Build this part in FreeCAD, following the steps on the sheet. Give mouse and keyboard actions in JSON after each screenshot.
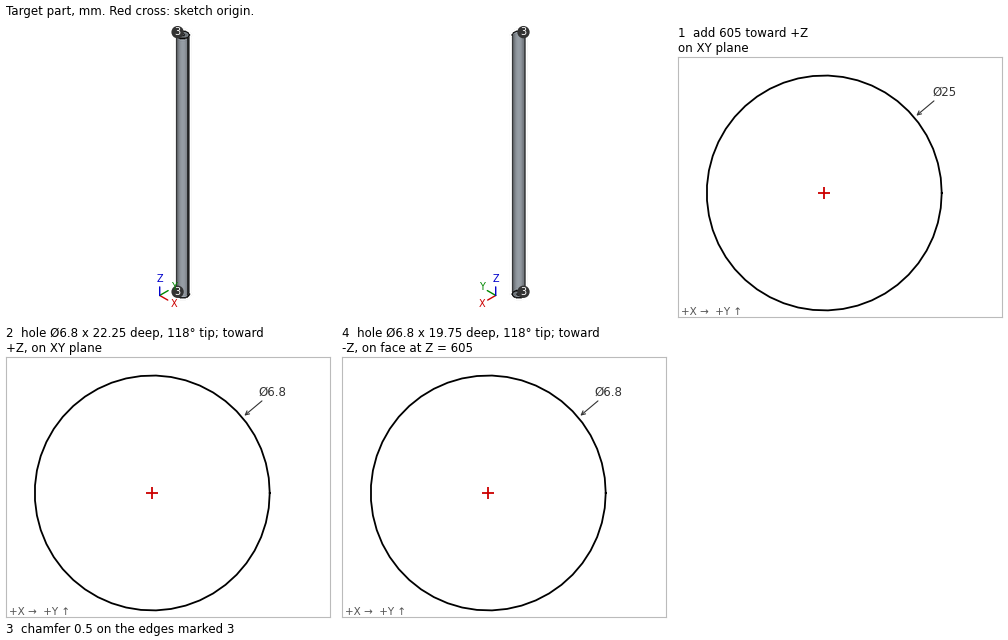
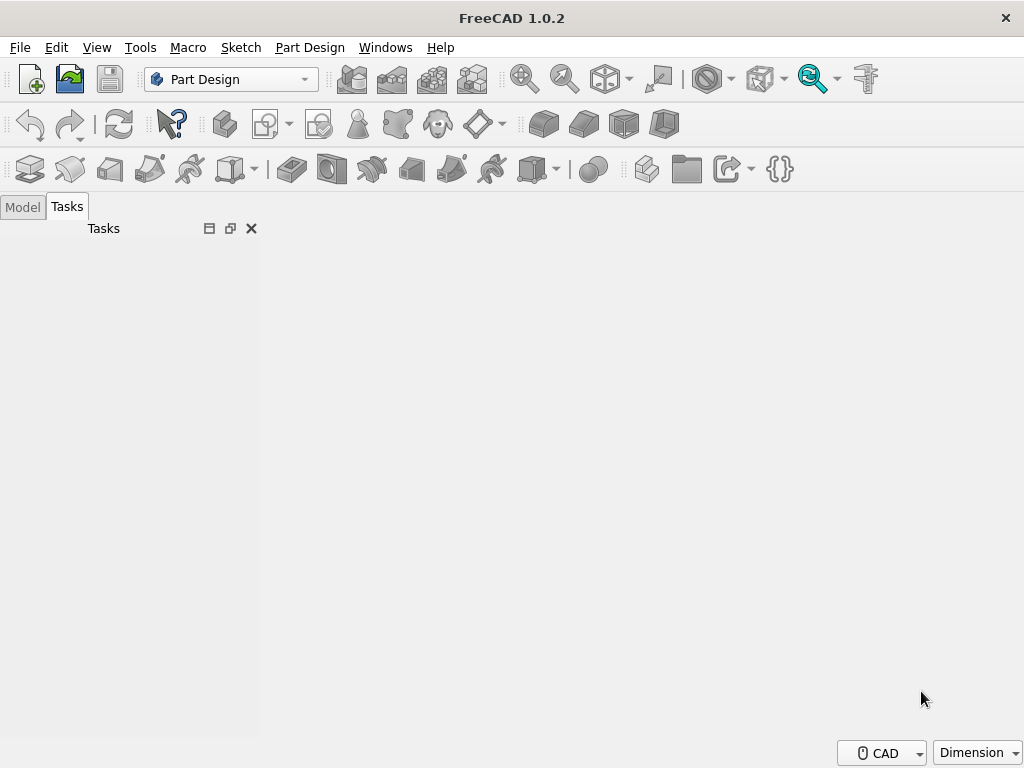
{"action": "left_click", "coordinate": [30, 80]}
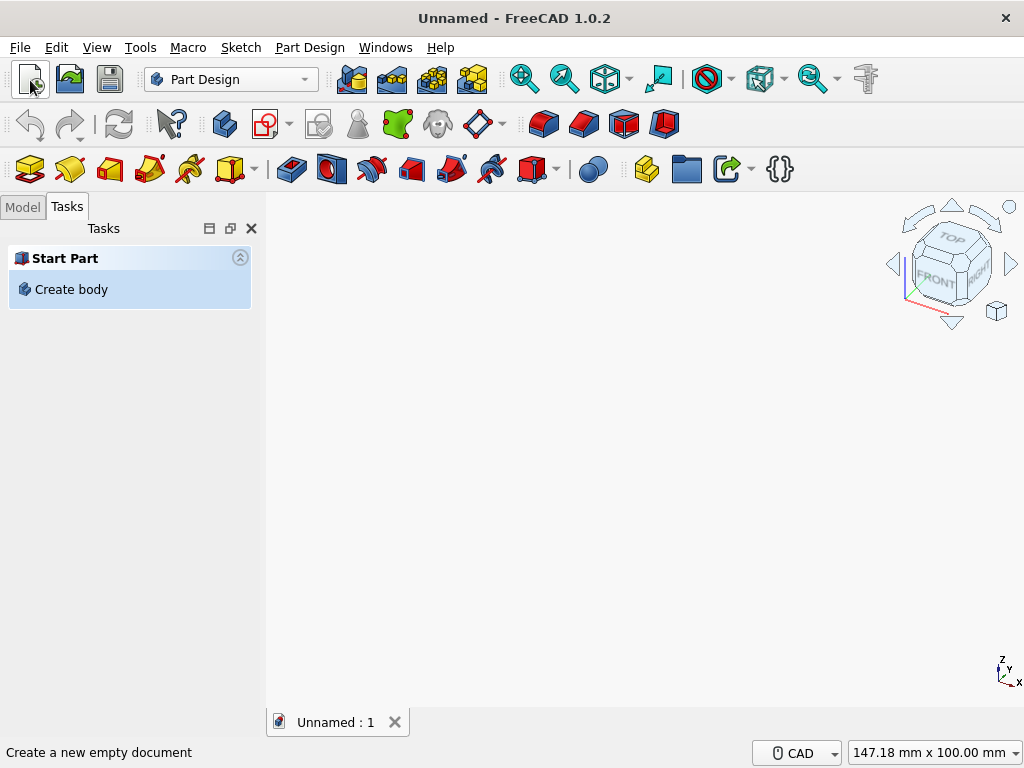
{"action": "left_click", "coordinate": [266, 124]}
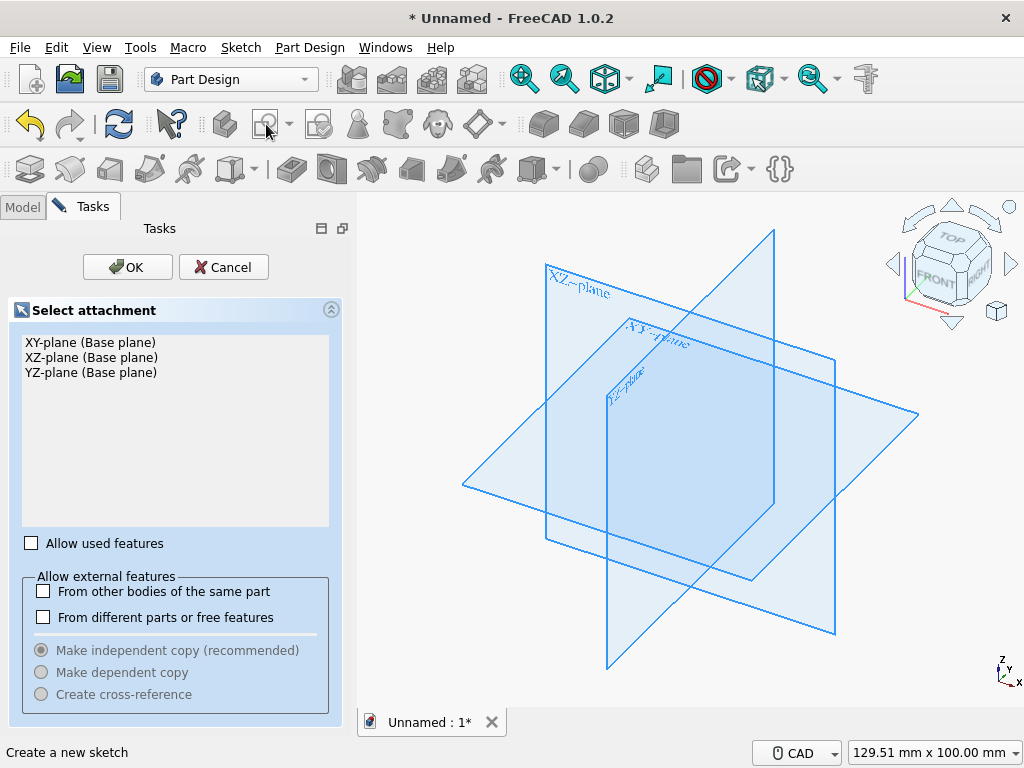
{"action": "left_click", "coordinate": [82, 342]}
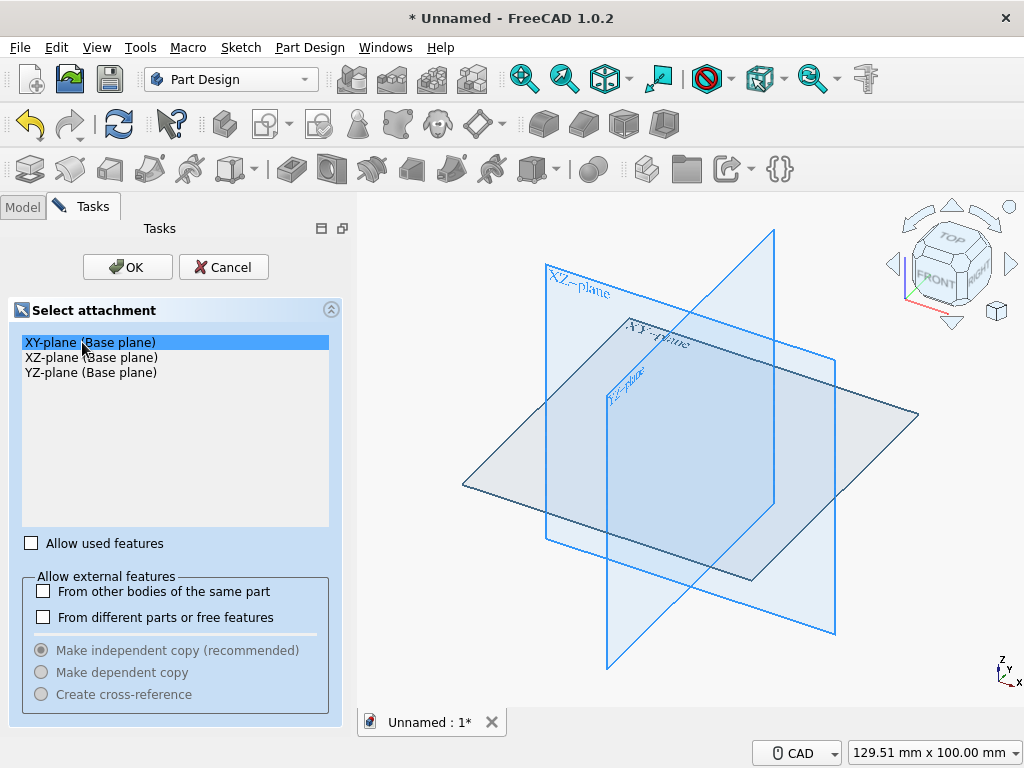
{"action": "left_click", "coordinate": [128, 267]}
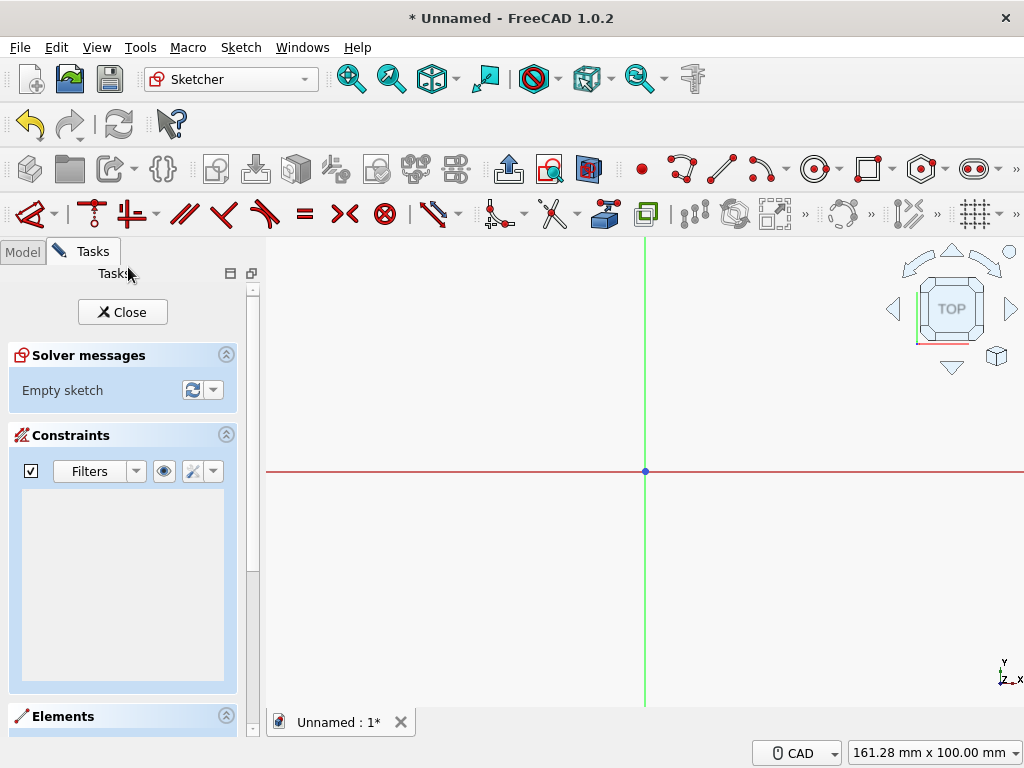
{"action": "scroll", "coordinate": [685, 472], "scroll_direction": "up", "scroll_amount": 5}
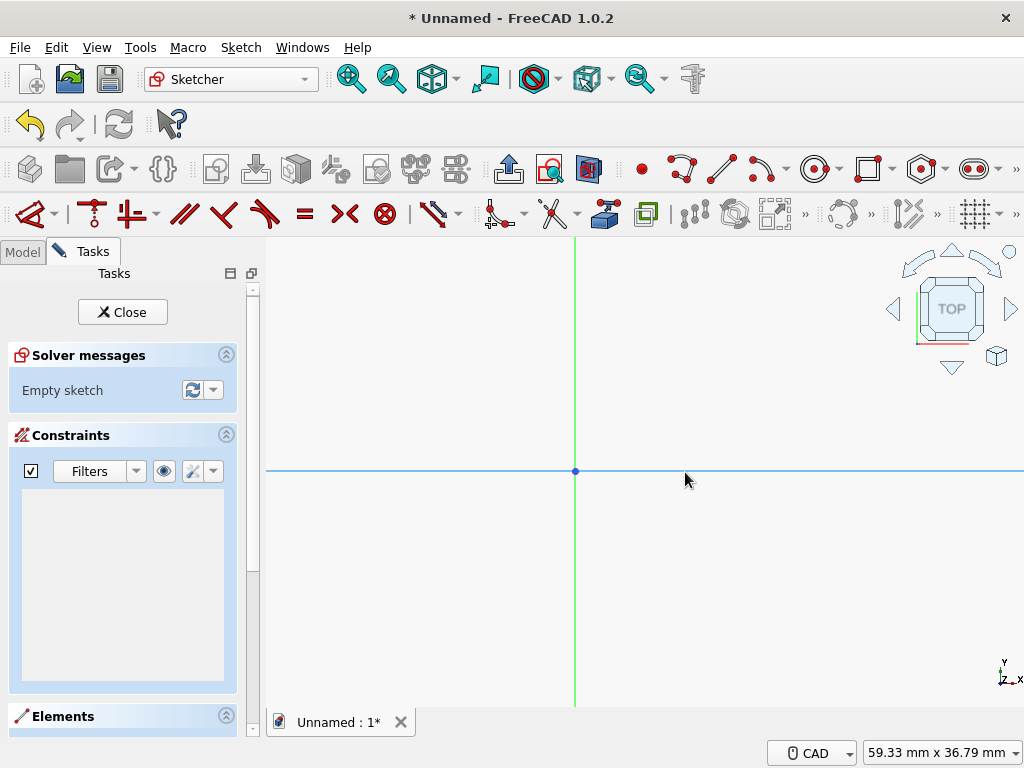
{"action": "key", "text": "g c"}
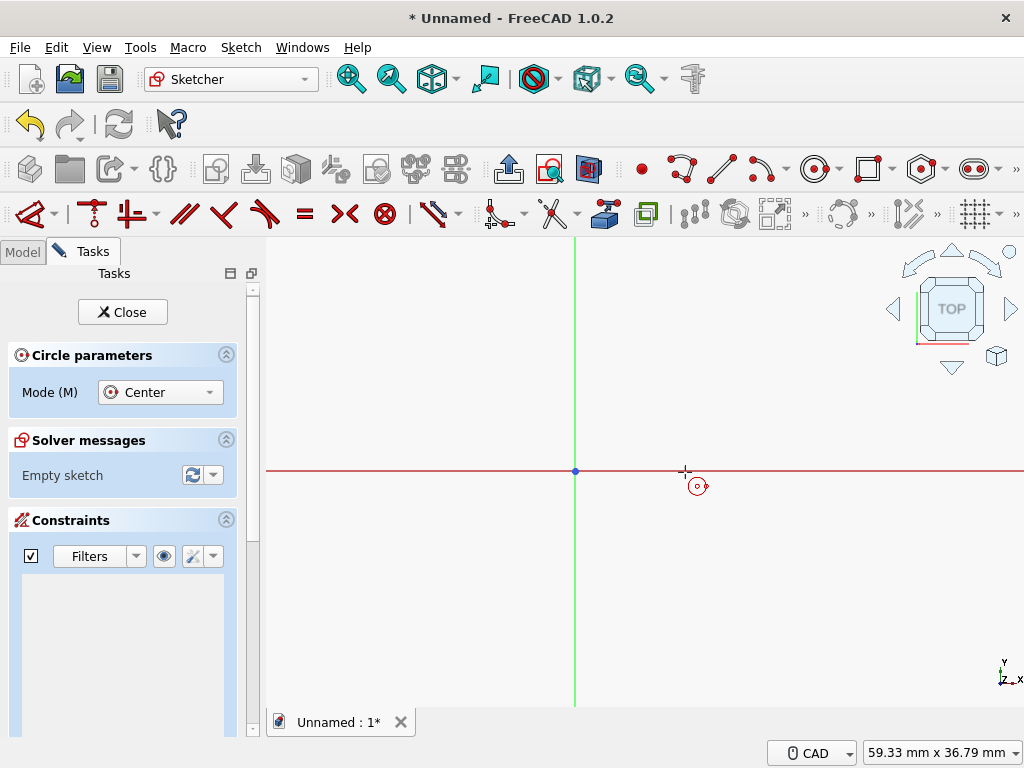
{"action": "left_click", "coordinate": [575, 471]}
{"action": "left_click", "coordinate": [688, 358]}
{"action": "key", "text": "Escape"}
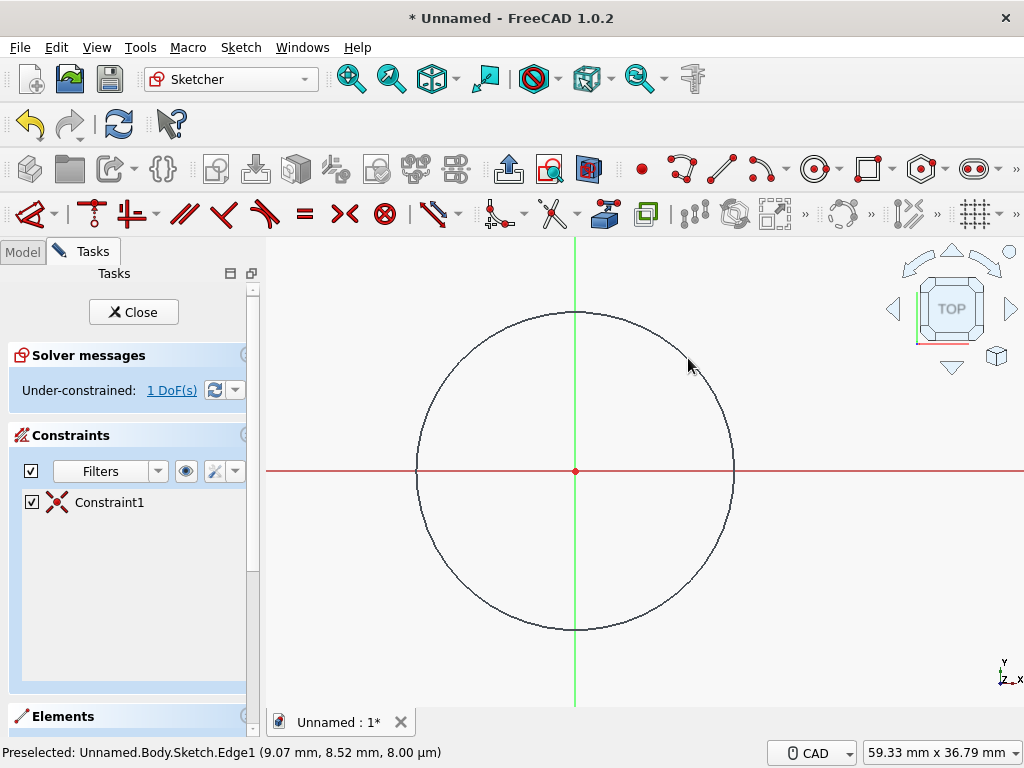
{"action": "left_click", "coordinate": [30, 214]}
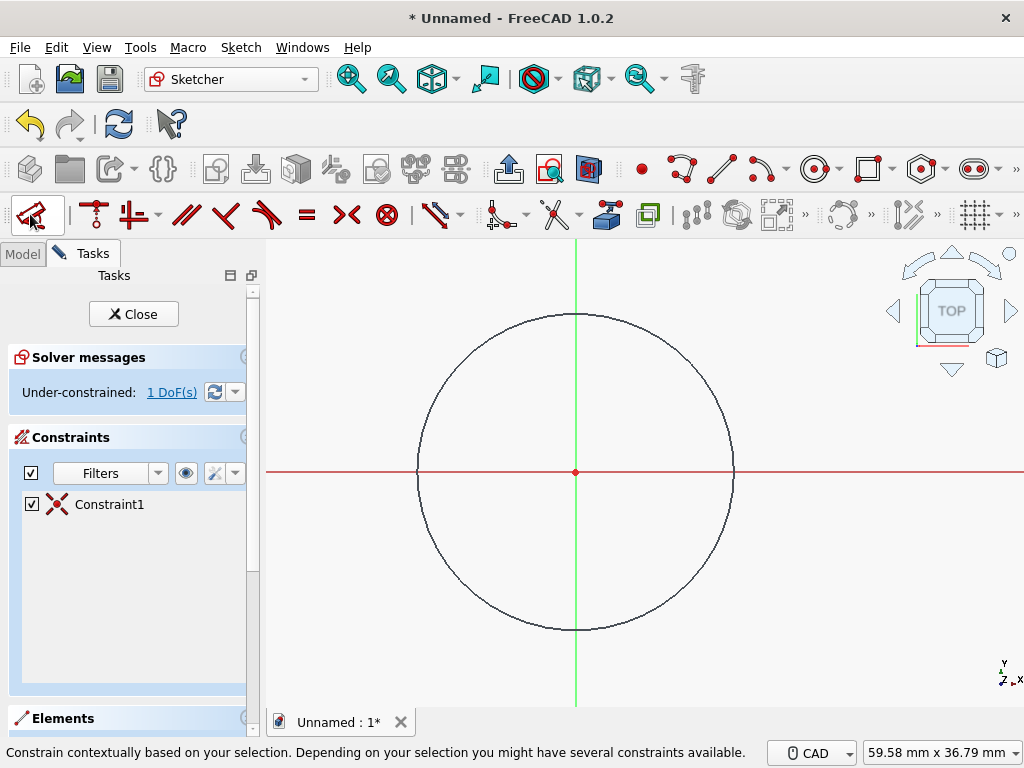
{"action": "left_click", "coordinate": [687, 360]}
{"action": "left_click", "coordinate": [710, 337]}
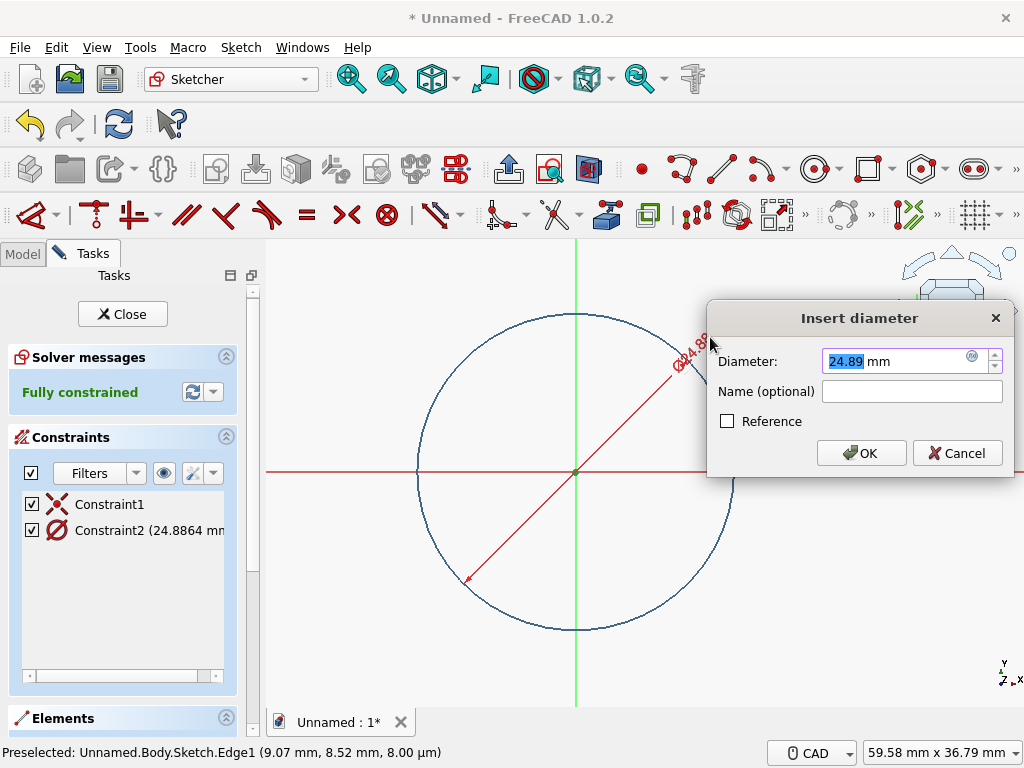
{"action": "type", "text": "25"}
{"action": "key", "text": "Return"}
{"action": "key", "text": "Escape"}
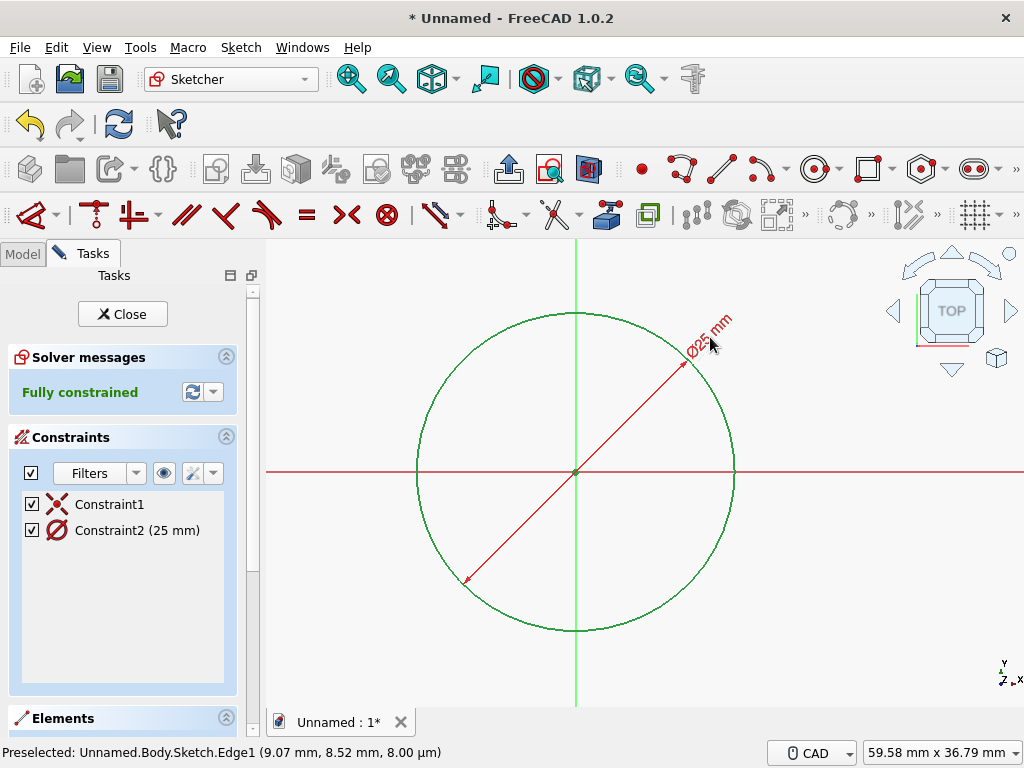
{"action": "left_click", "coordinate": [123, 314]}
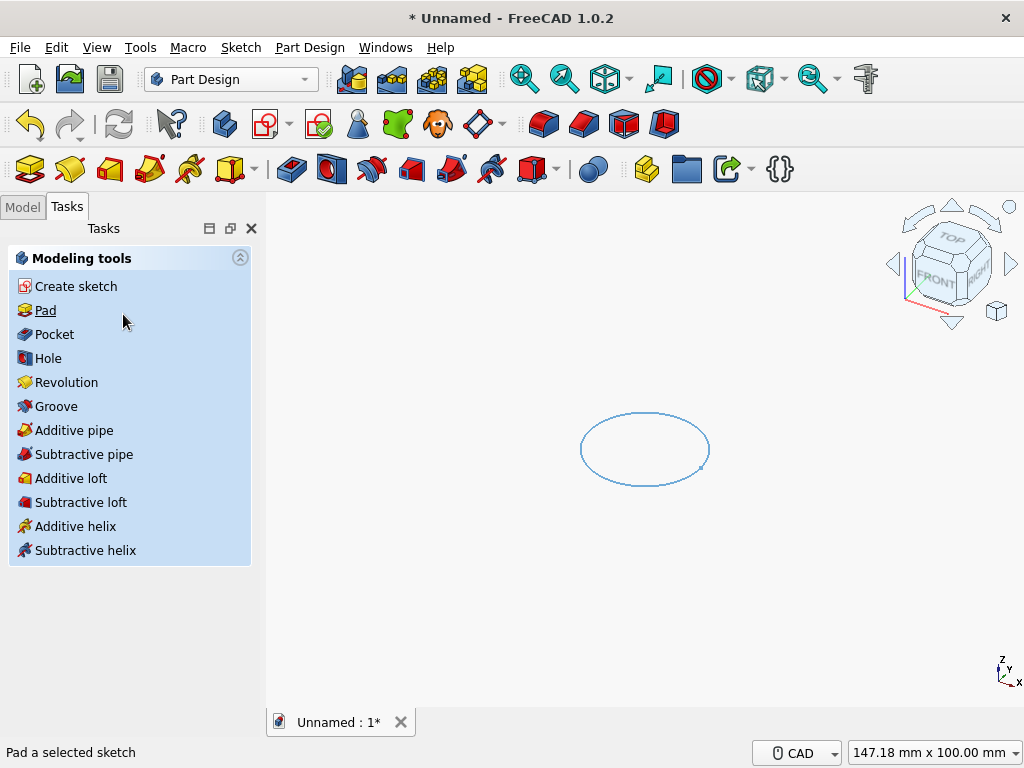
{"action": "left_click", "coordinate": [30, 170]}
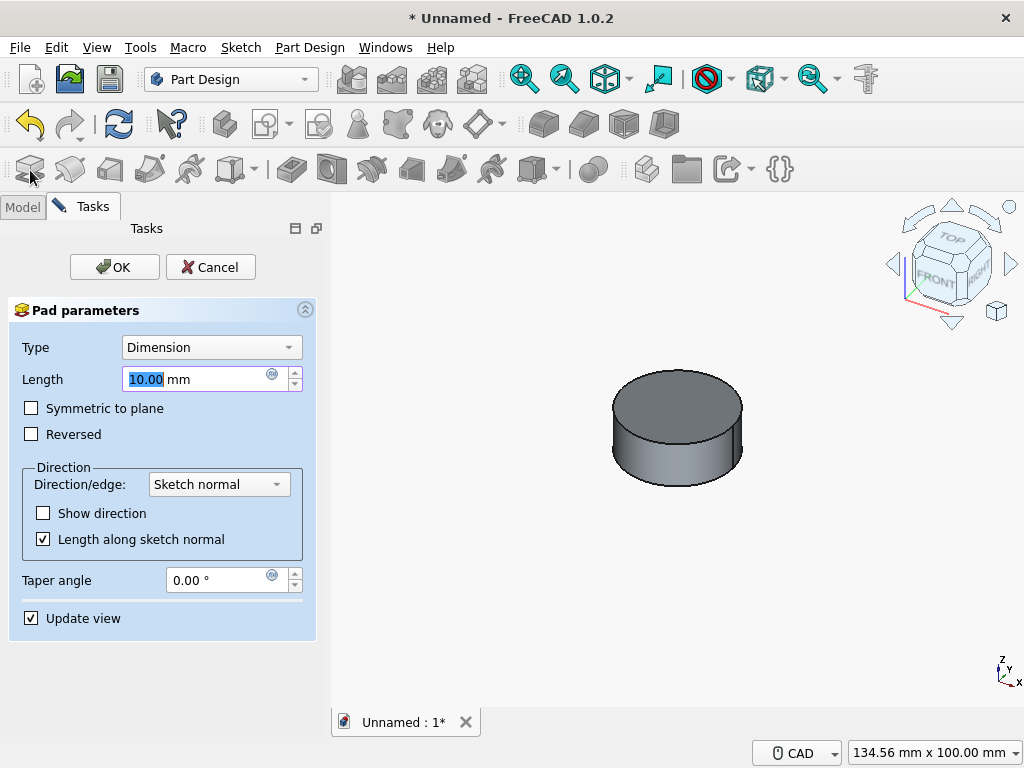
{"action": "type", "text": "605"}
{"action": "key", "text": "Tab"}